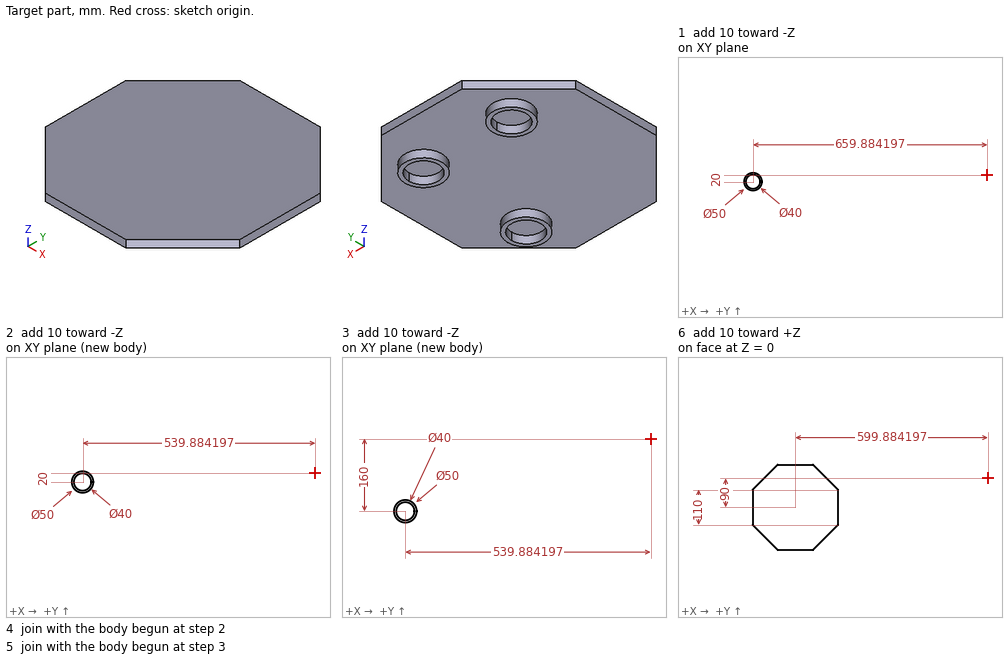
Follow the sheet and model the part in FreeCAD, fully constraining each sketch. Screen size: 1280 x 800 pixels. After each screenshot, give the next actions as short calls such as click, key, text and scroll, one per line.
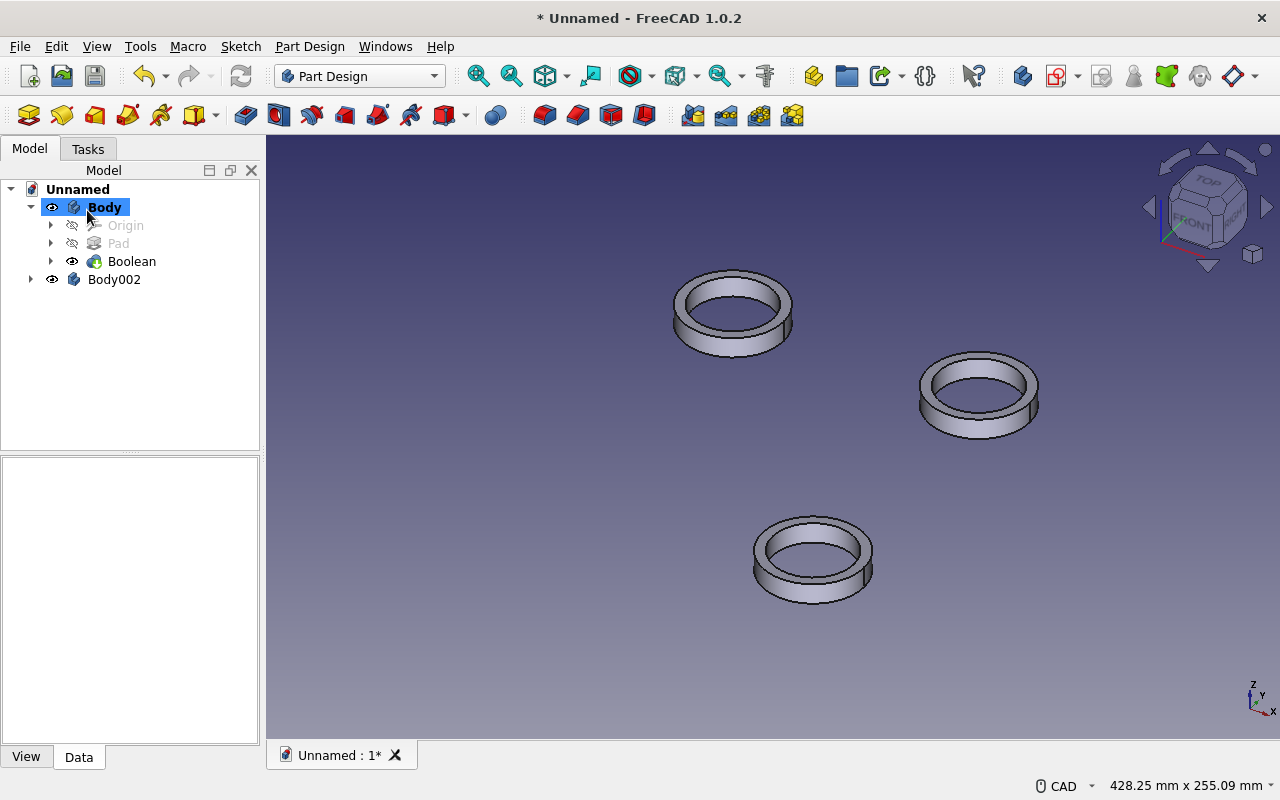
key(v)
key(f)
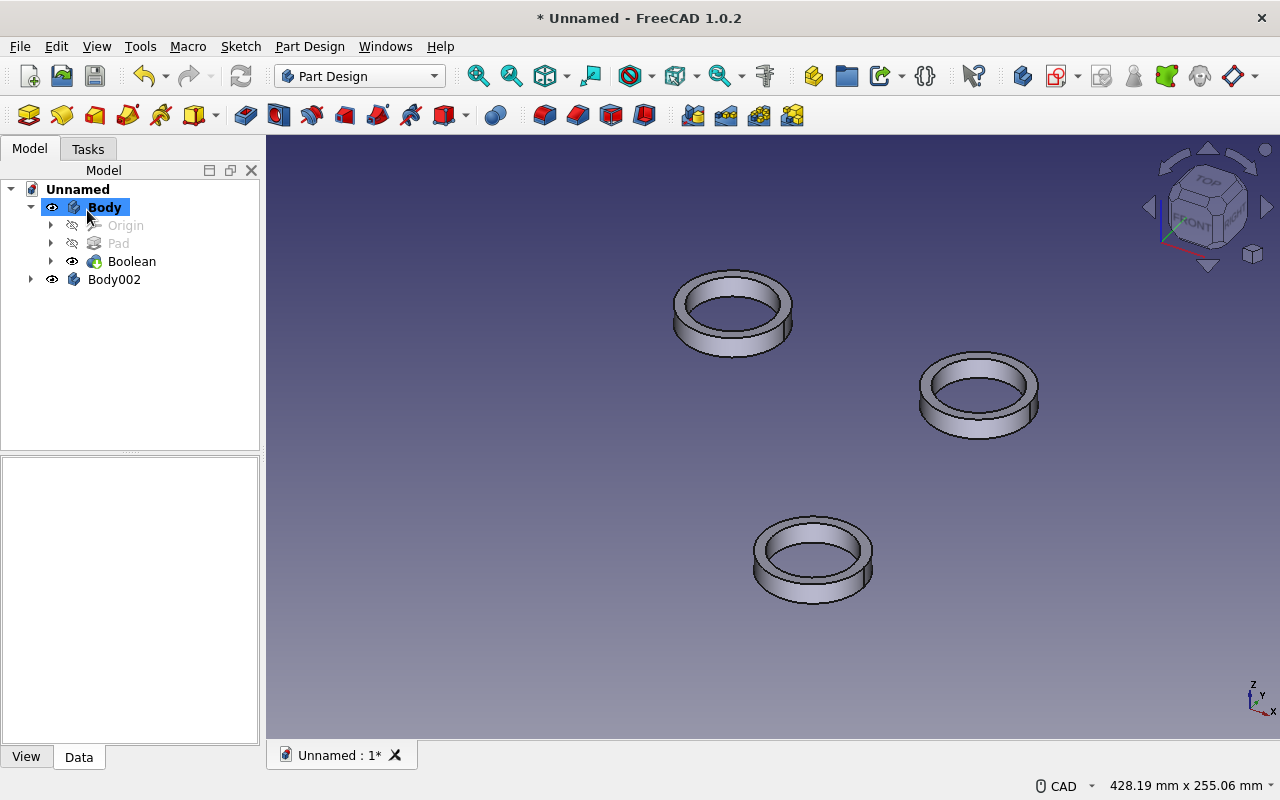
click(97, 279)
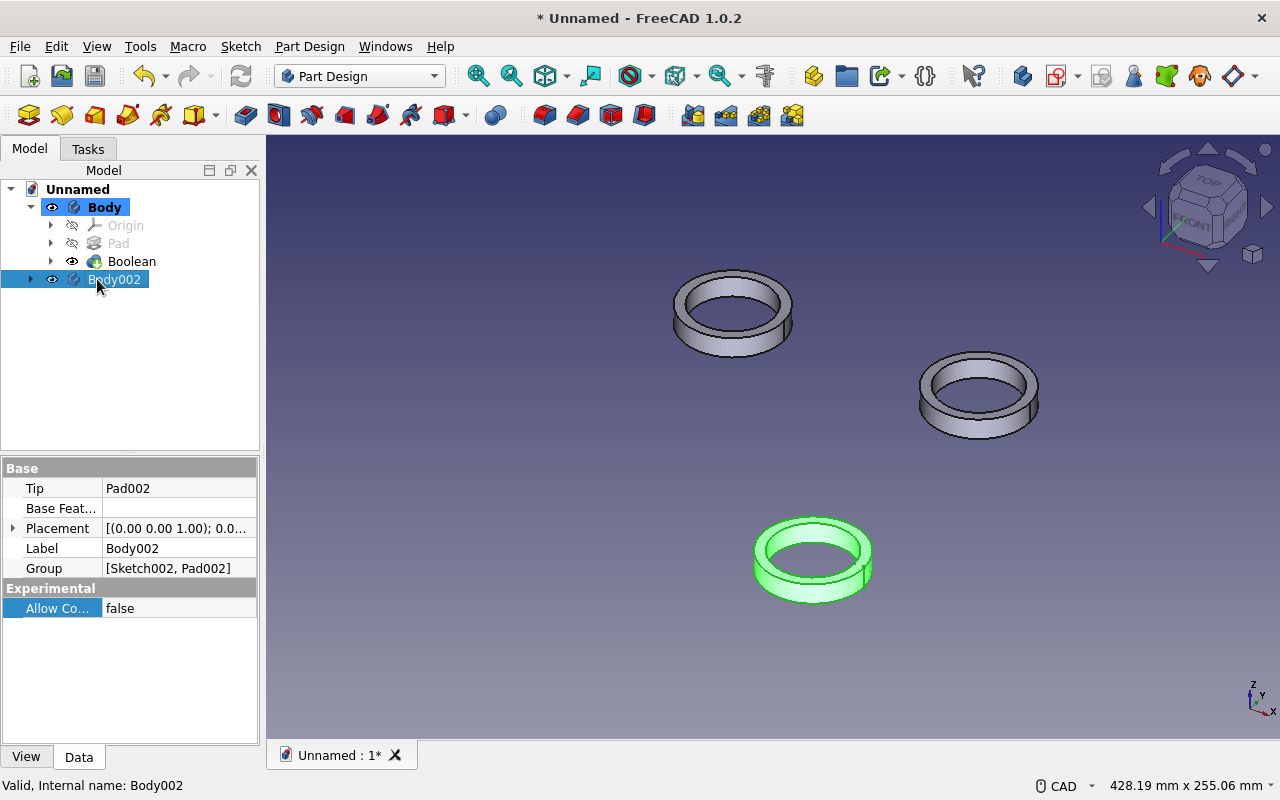
click(496, 116)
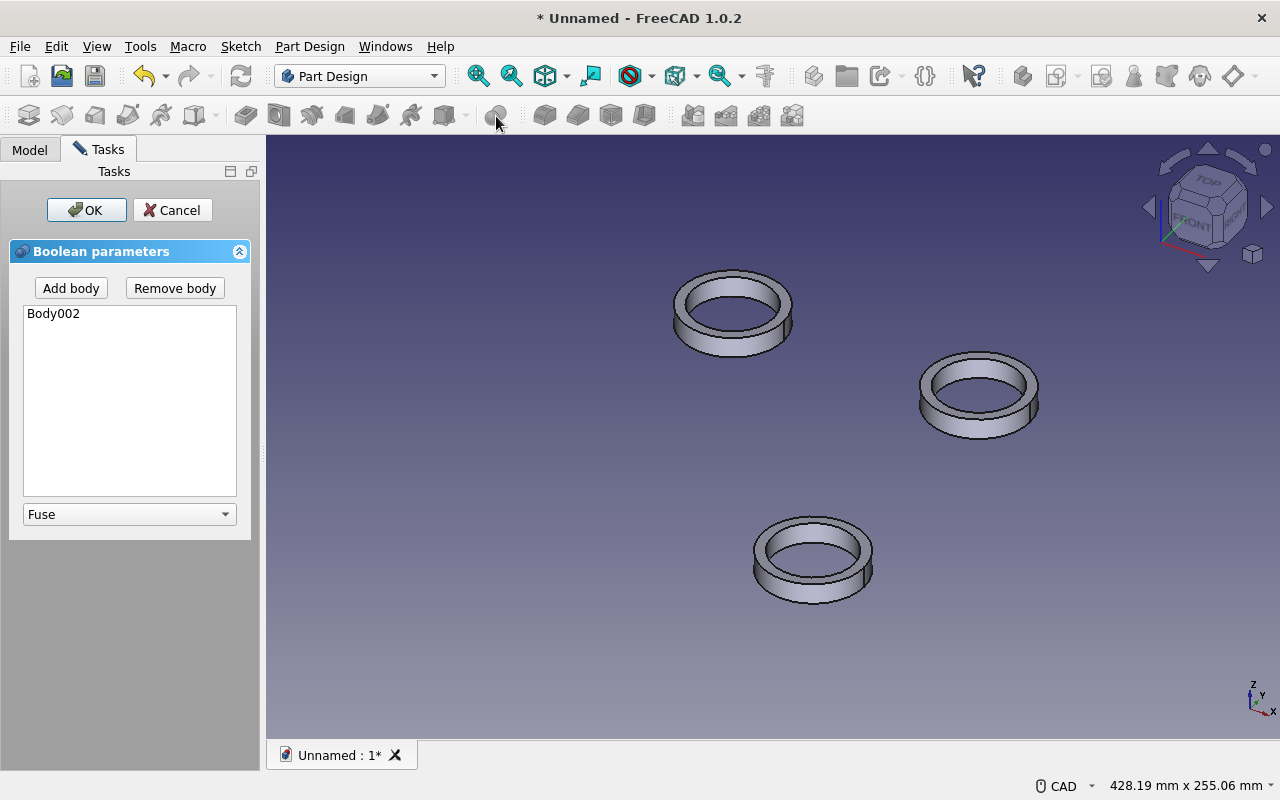
click(87, 210)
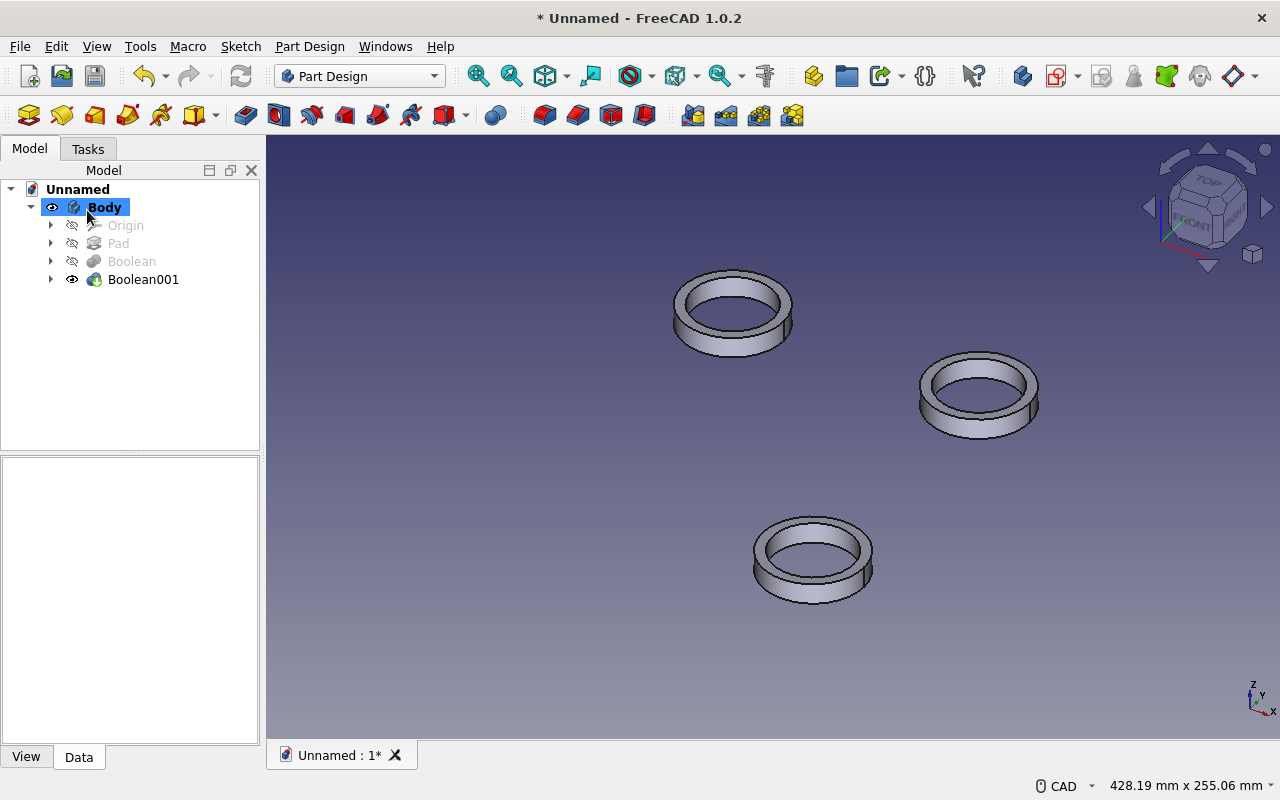
scroll(968, 415, up, 4)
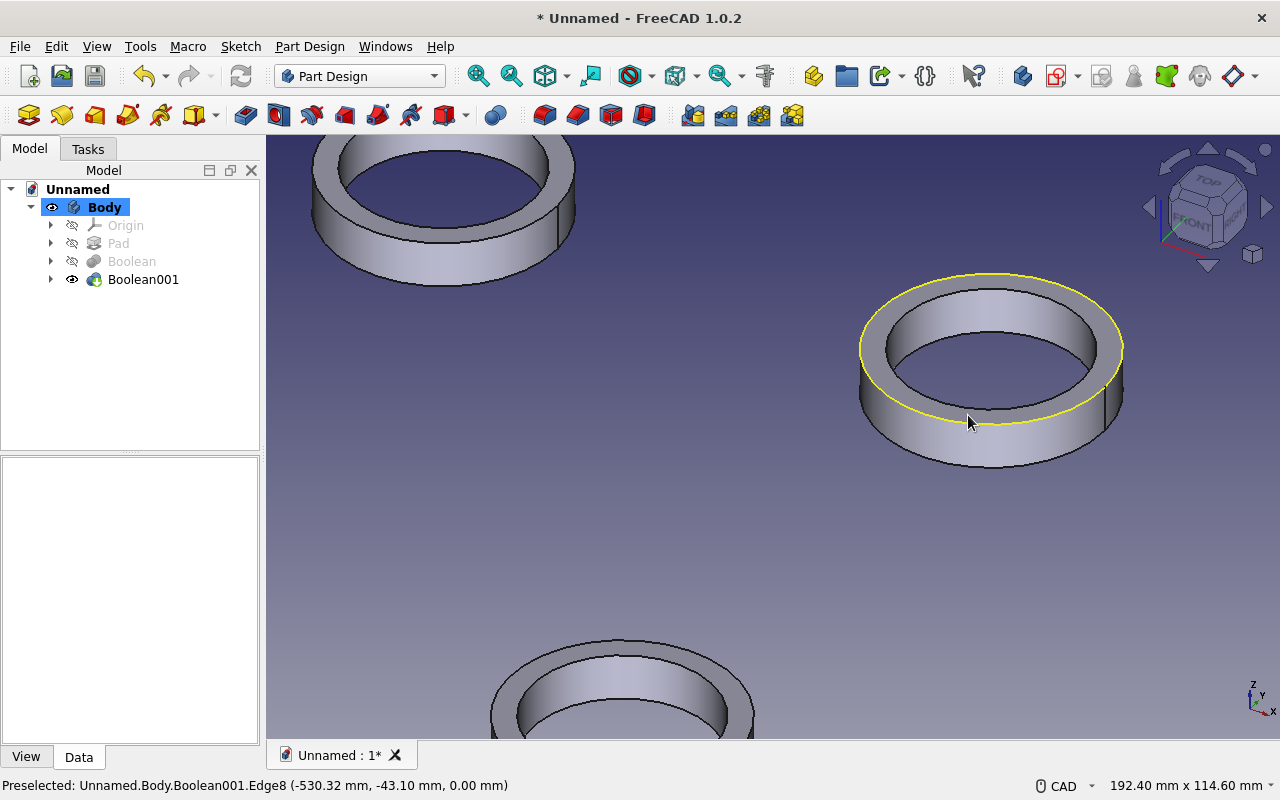
click(1080, 303)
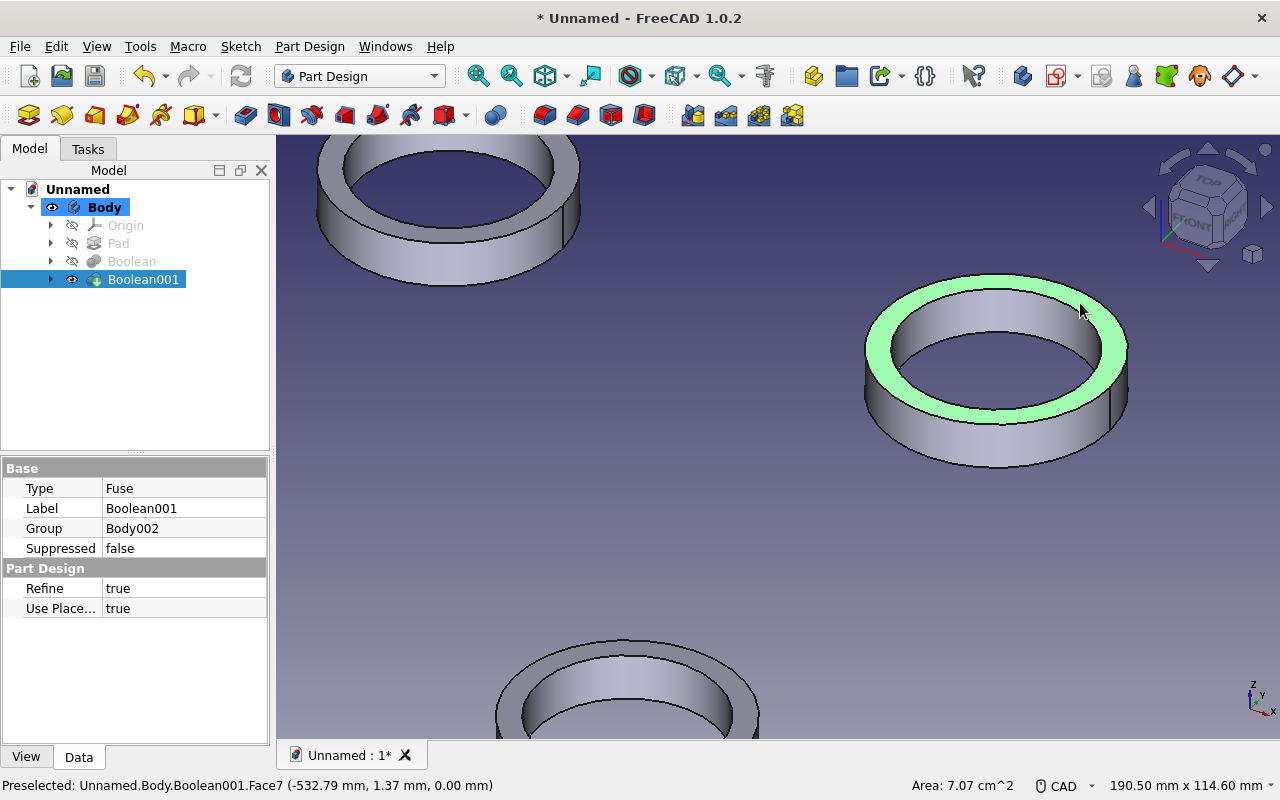
click(1056, 76)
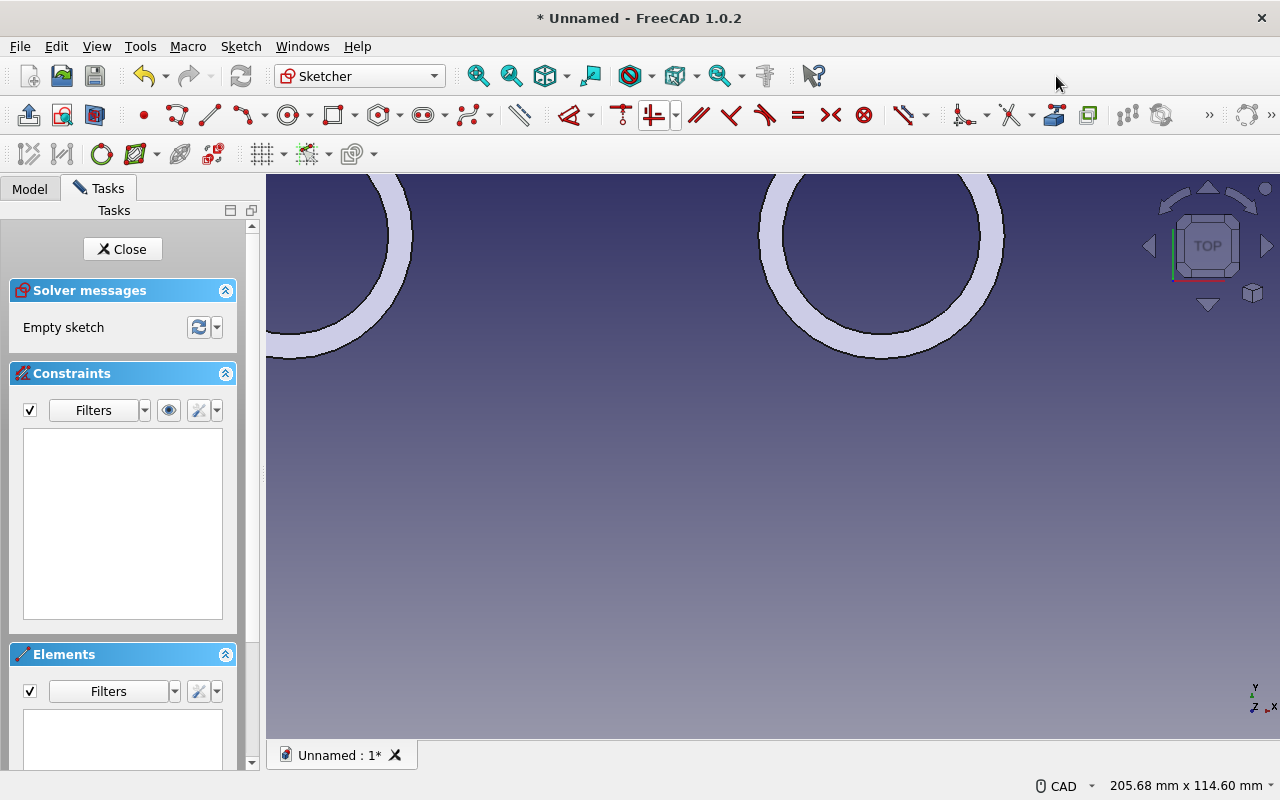
scroll(756, 403, down, 6)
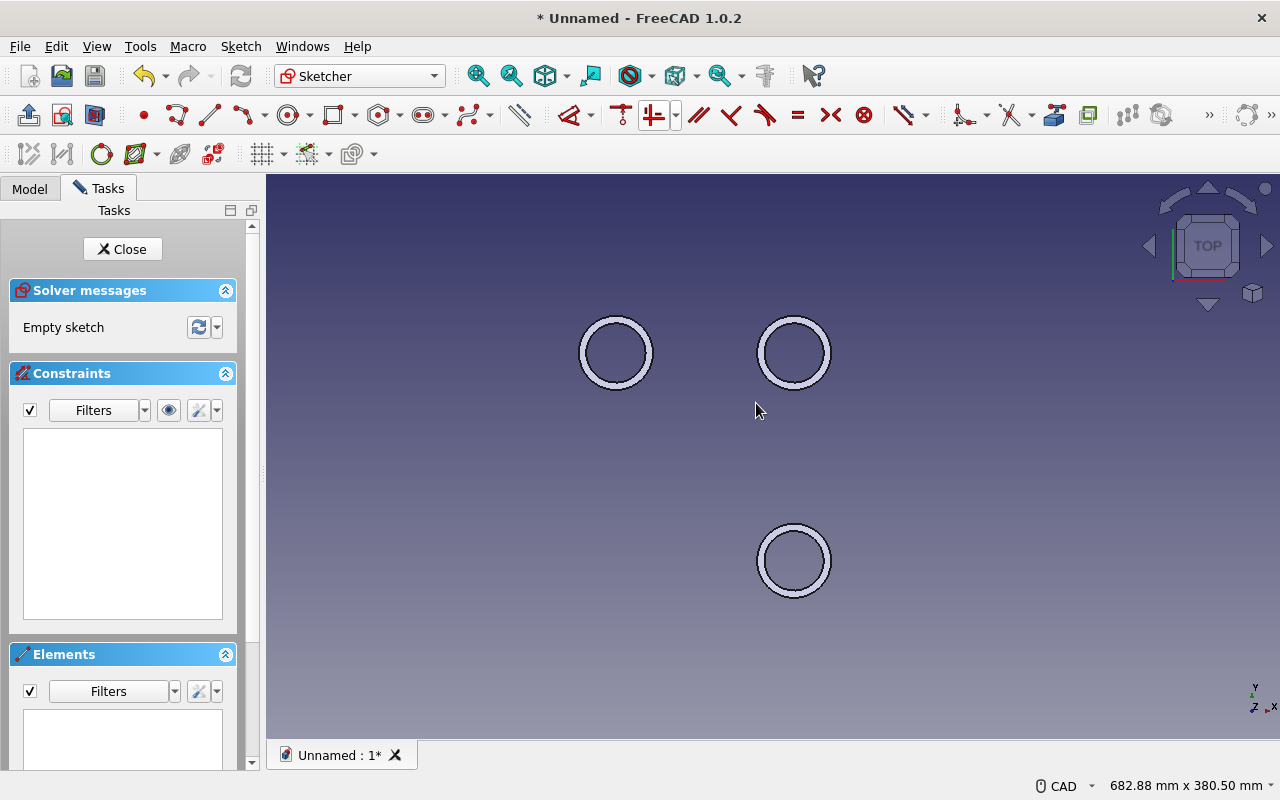
key(g)
key(p)
key(8)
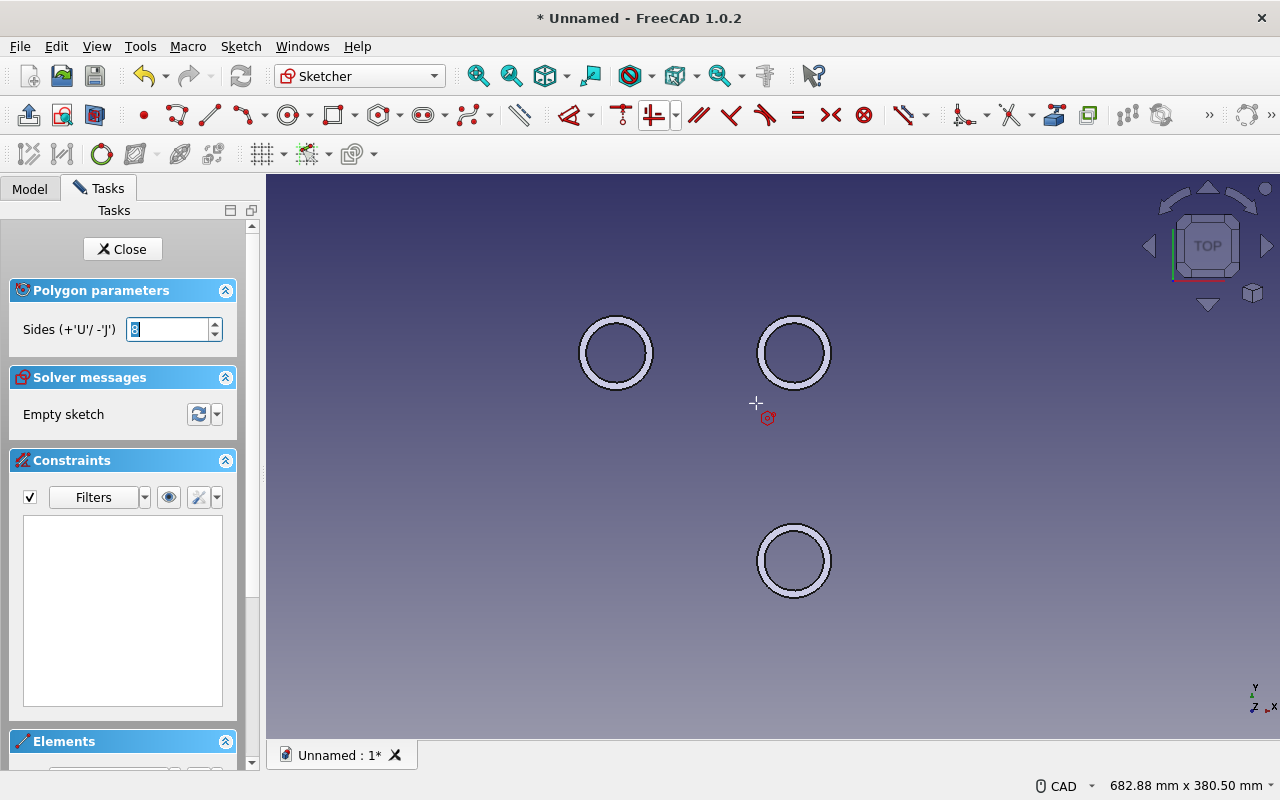
click(705, 457)